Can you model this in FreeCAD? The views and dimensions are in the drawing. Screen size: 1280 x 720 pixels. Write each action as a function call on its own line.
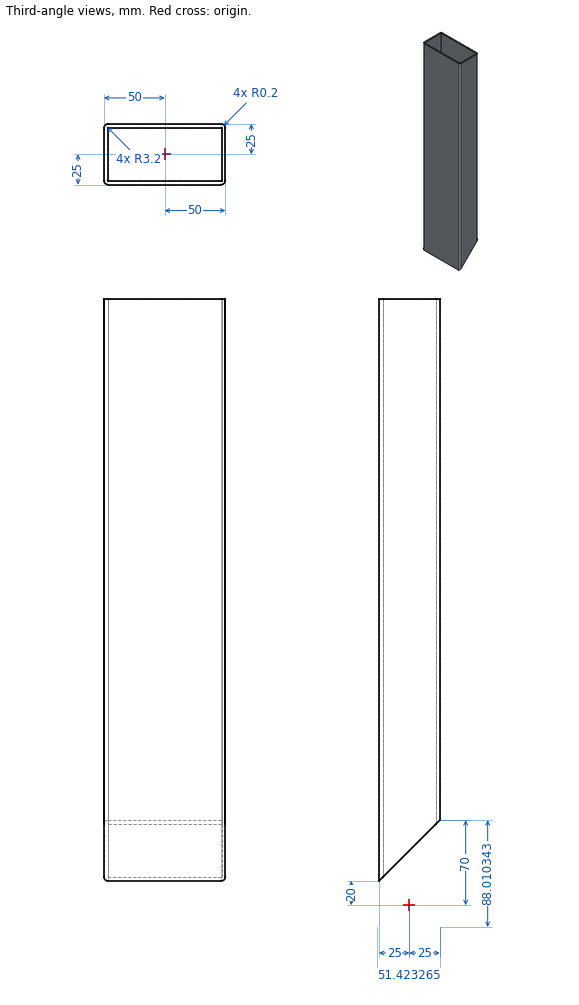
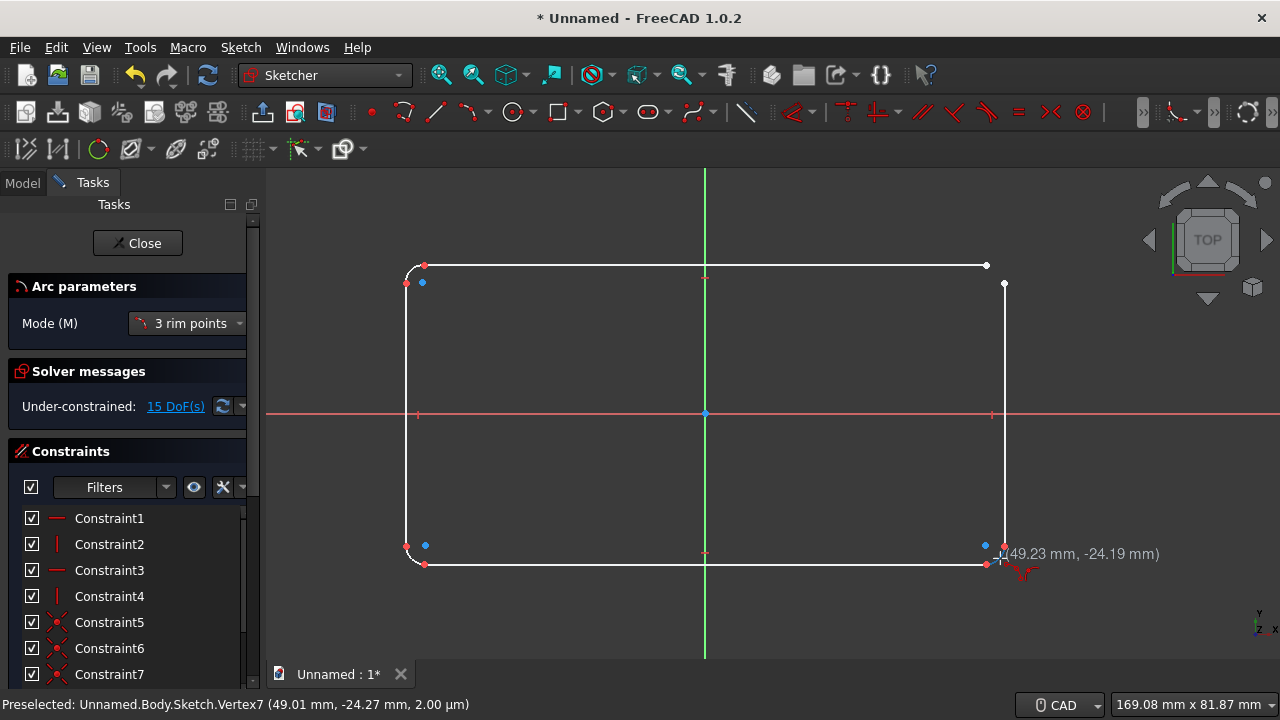
click(1005, 284)
click(986, 265)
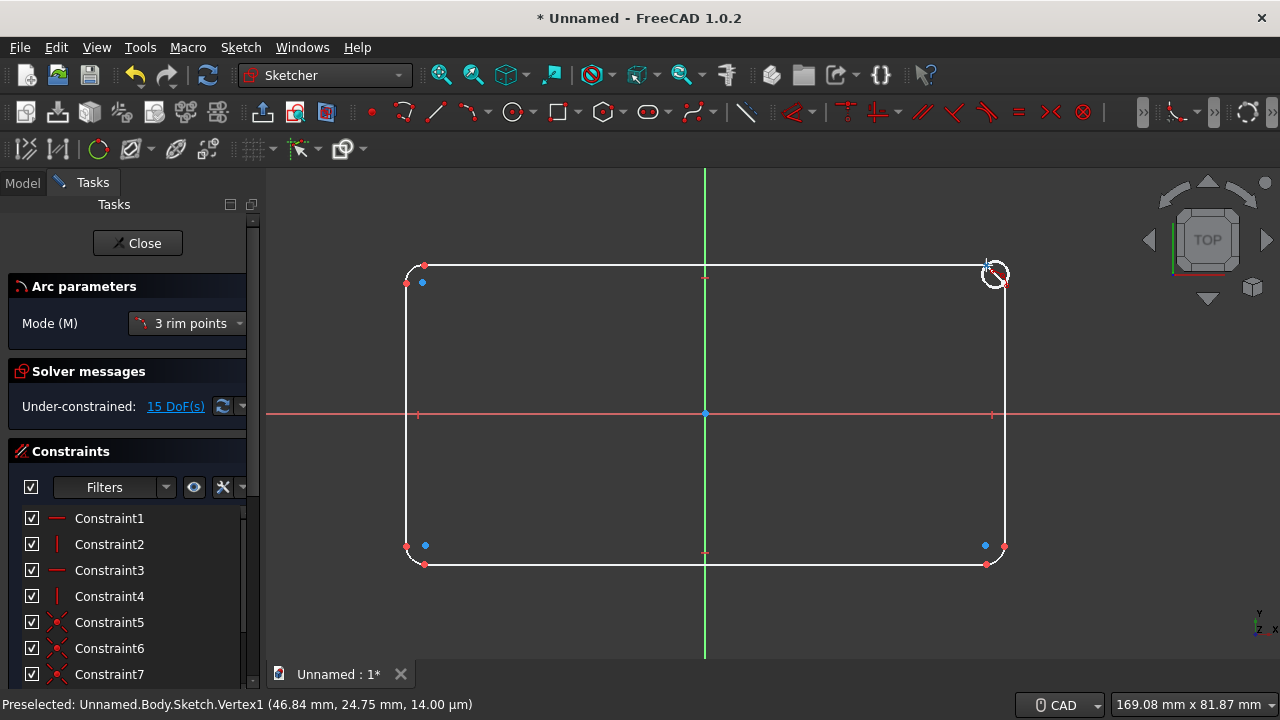
scroll(1000, 269, up, 6)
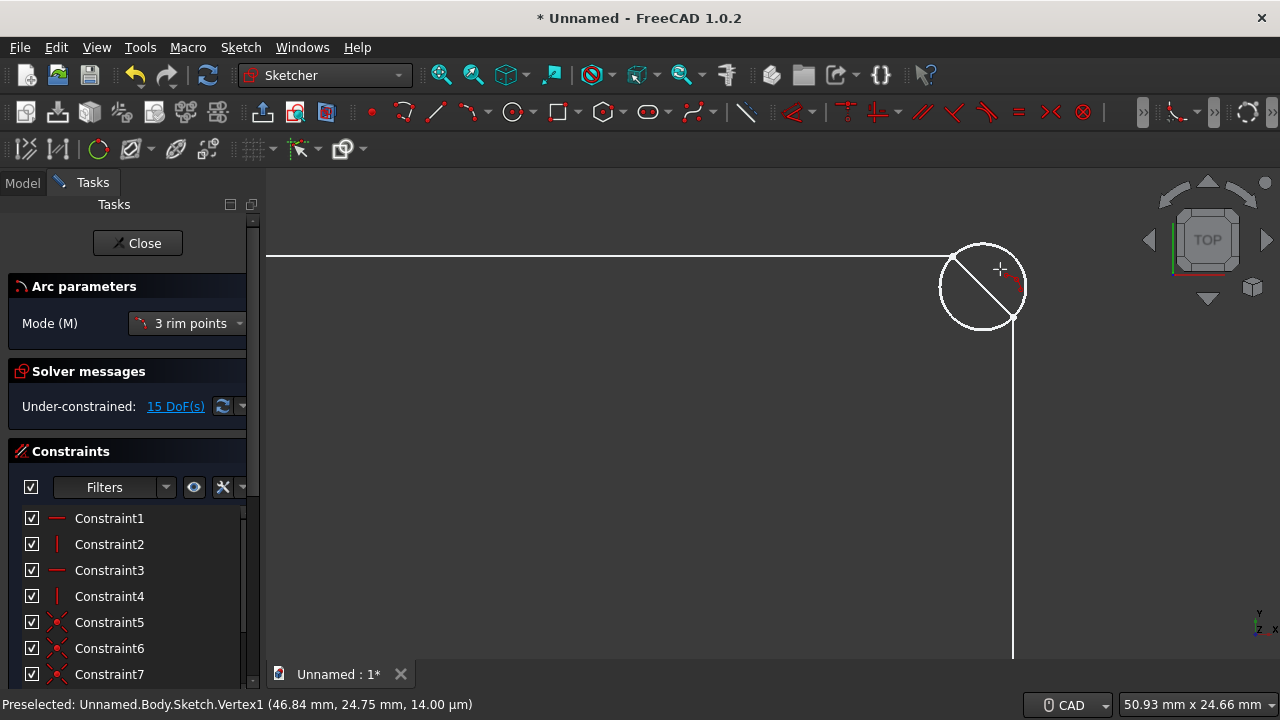
click(997, 270)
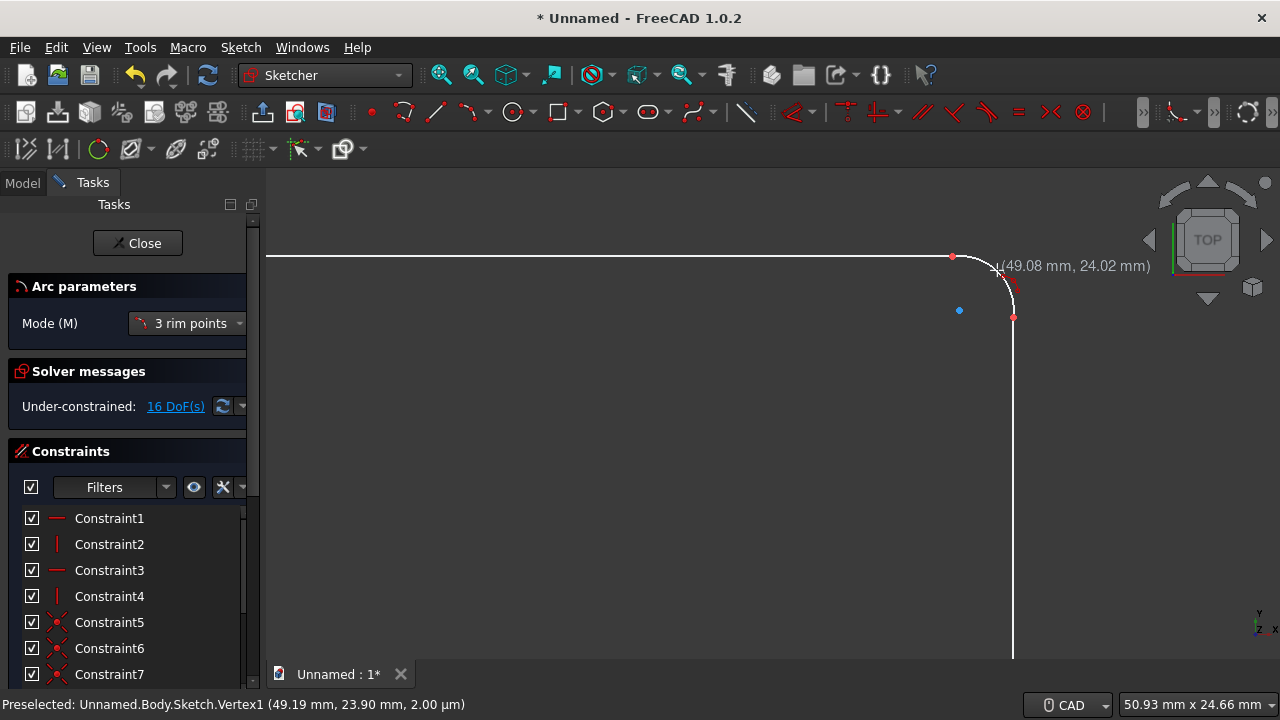
click(436, 112)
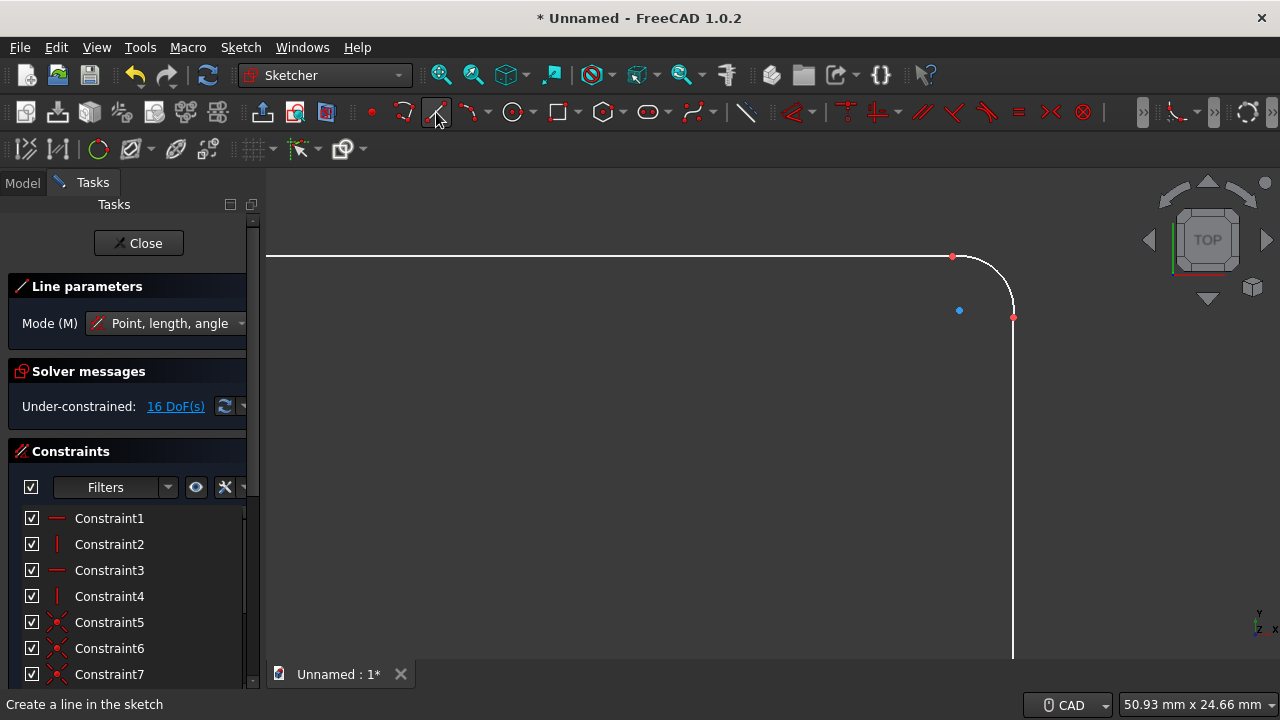
scroll(1000, 269, down, 6)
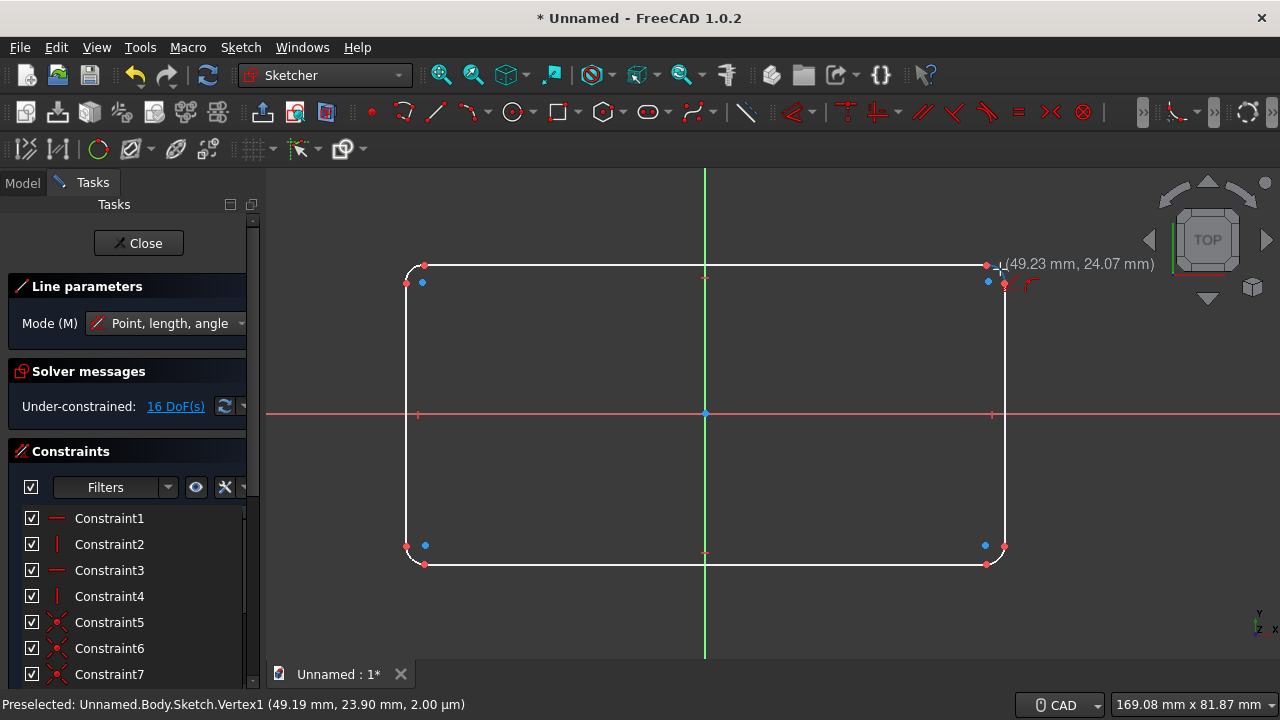
scroll(425, 282, up, 13)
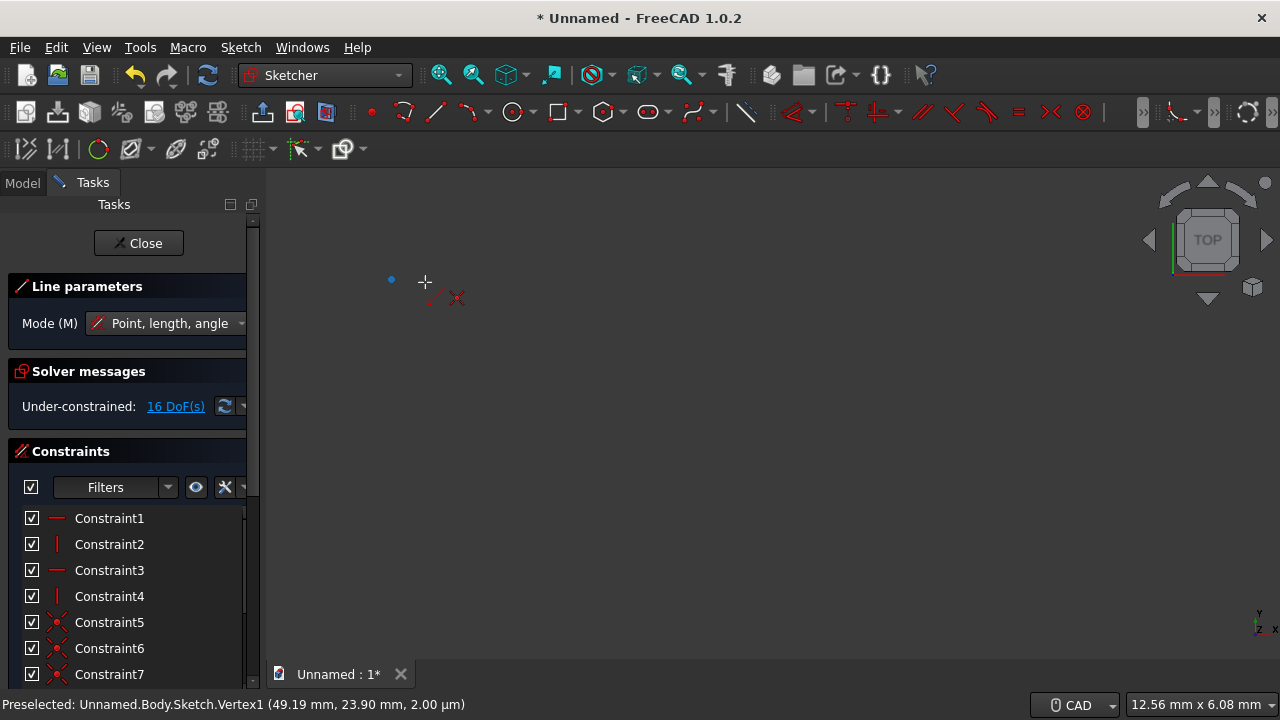
click(418, 277)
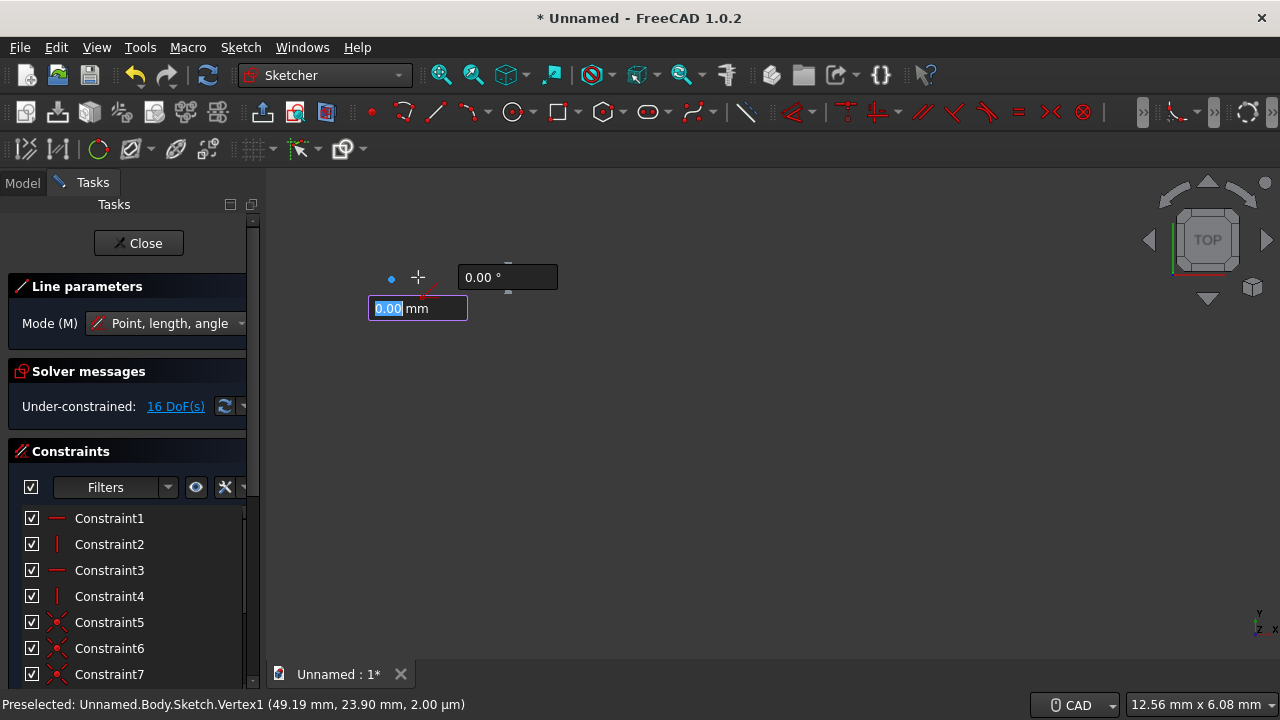
scroll(424, 282, down, 13)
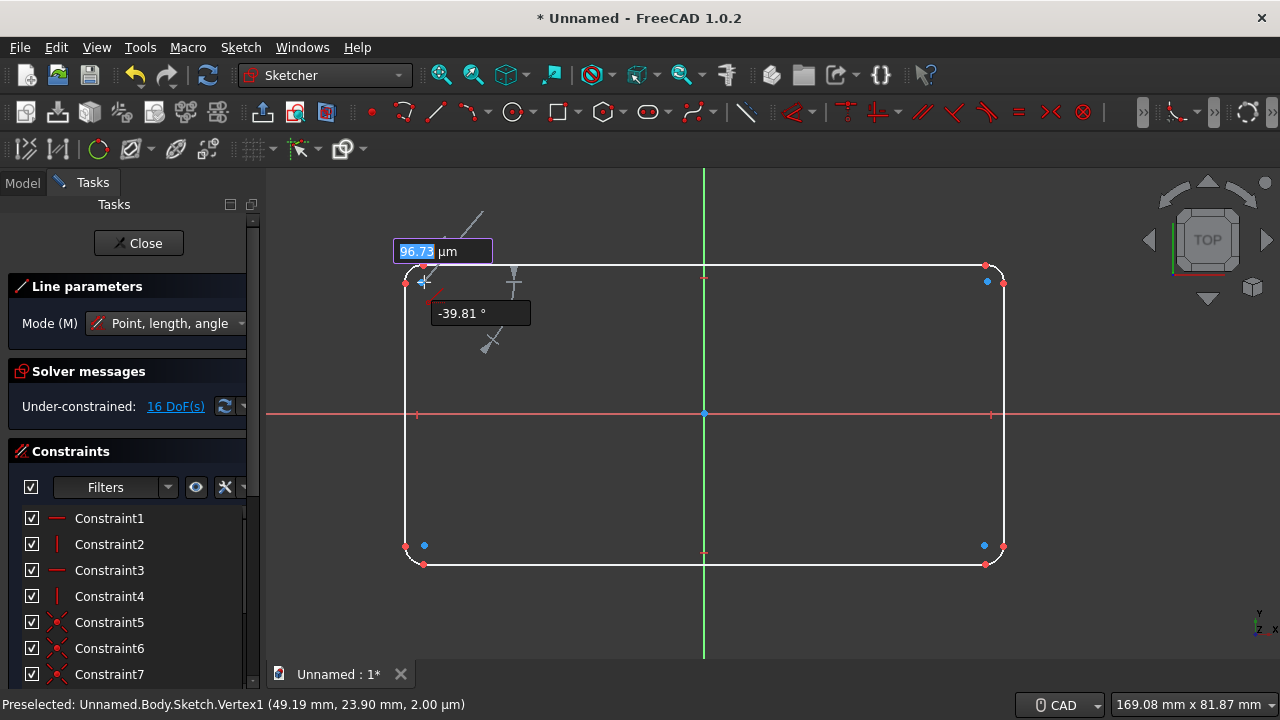
scroll(985, 282, up, 13)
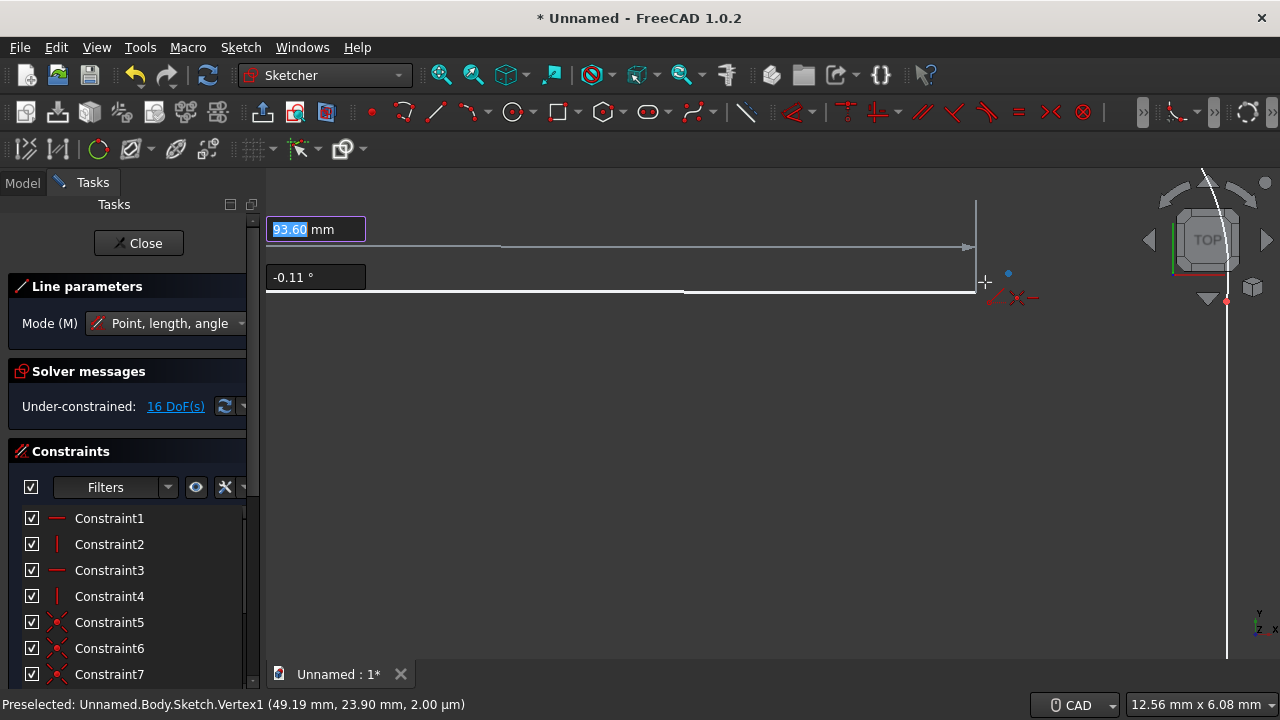
click(976, 277)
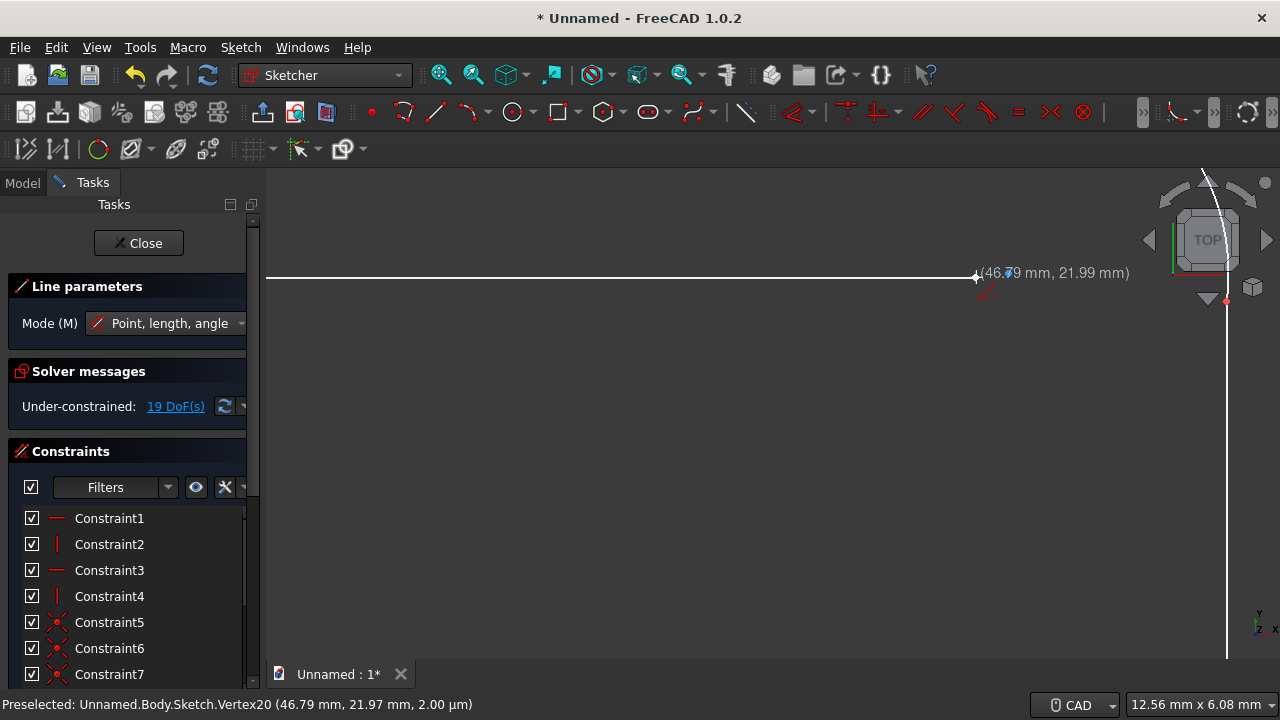
click(993, 293)